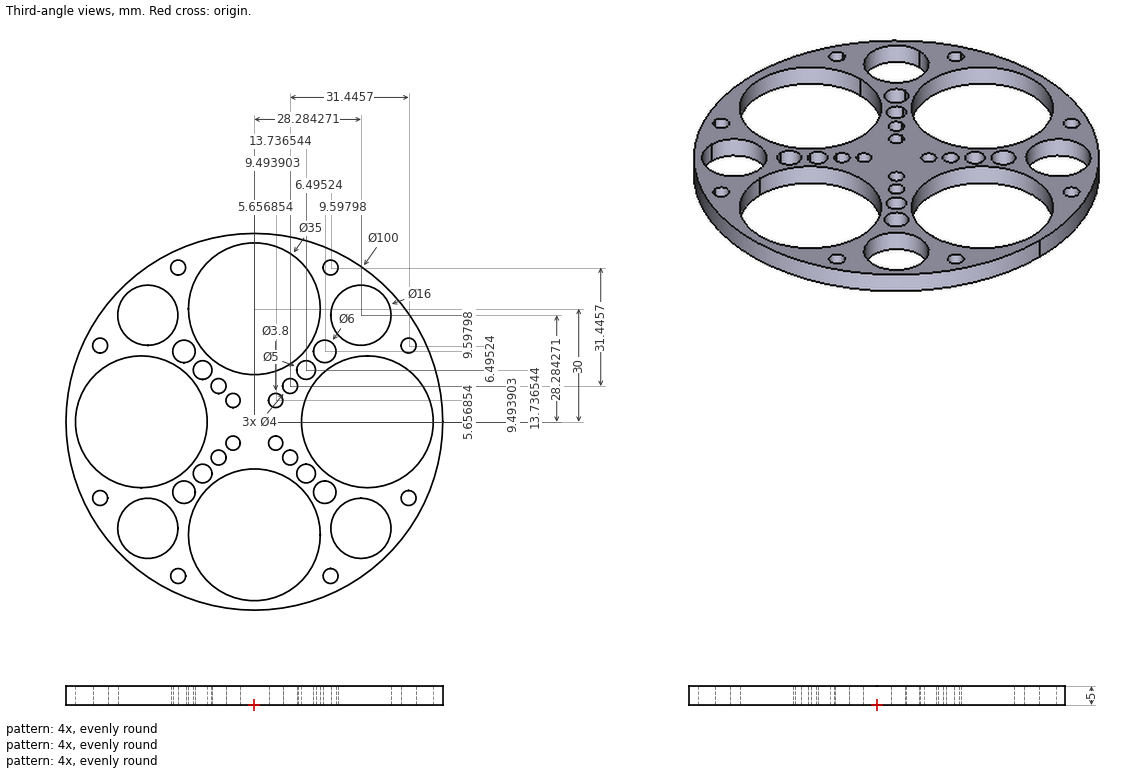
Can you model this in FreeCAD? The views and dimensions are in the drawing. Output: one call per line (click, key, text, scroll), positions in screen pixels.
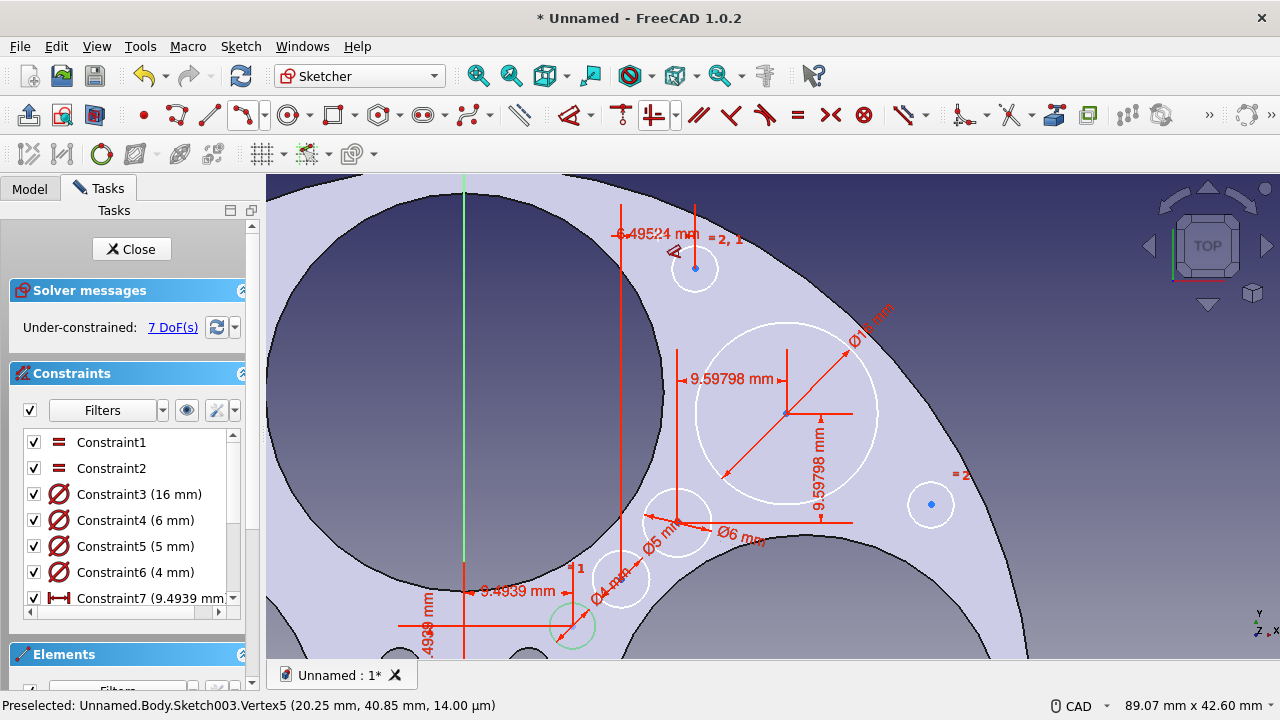
click(573, 626)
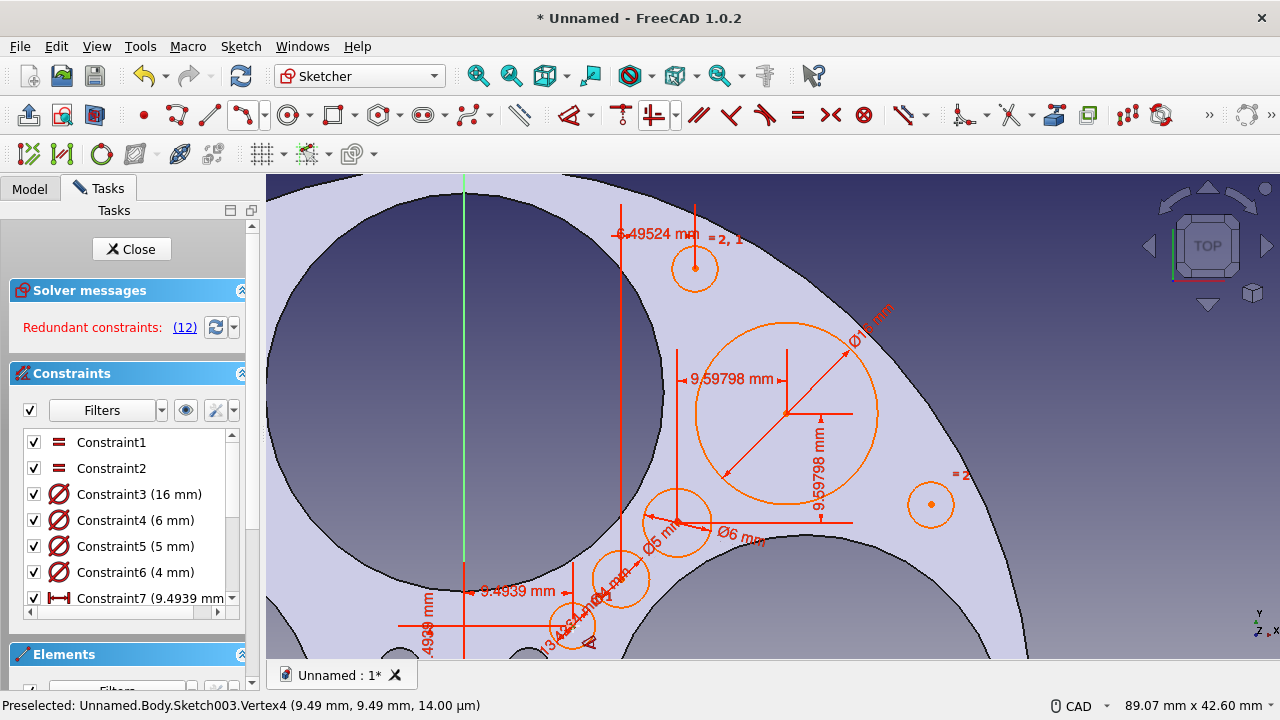
click(695, 269)
click(539, 448)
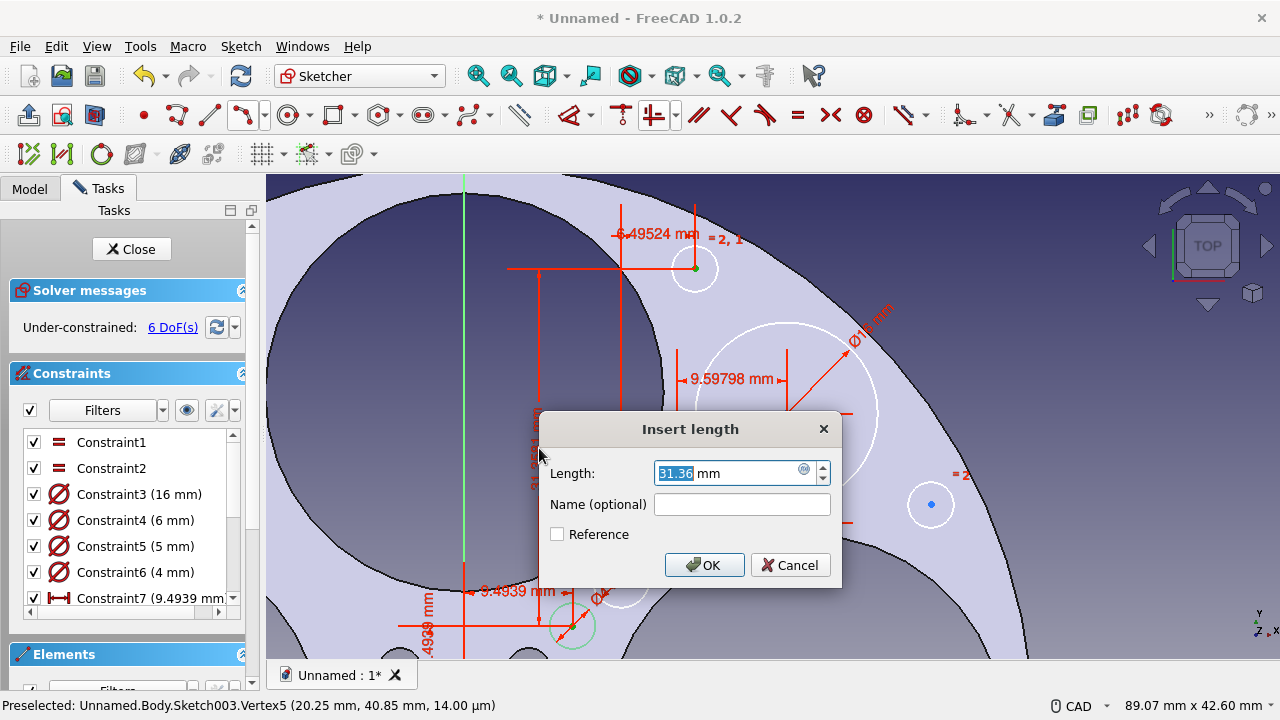
text(31.4457)
key(Return)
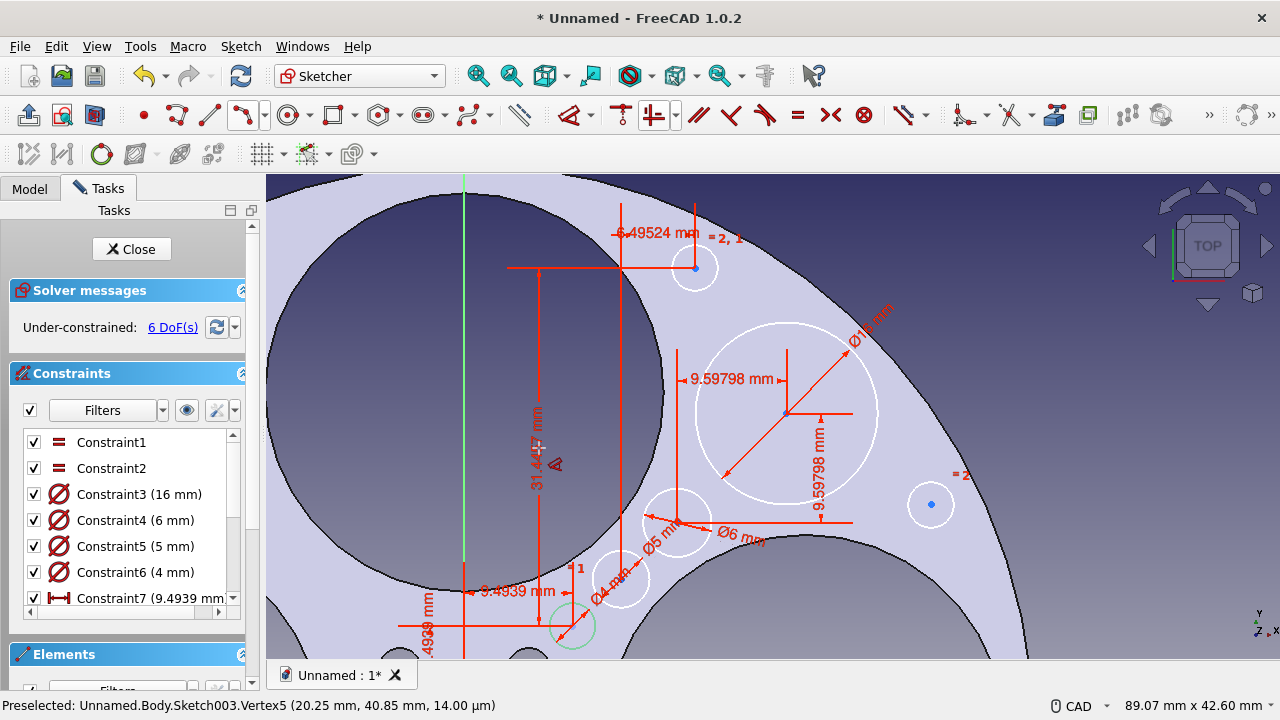
click(573, 626)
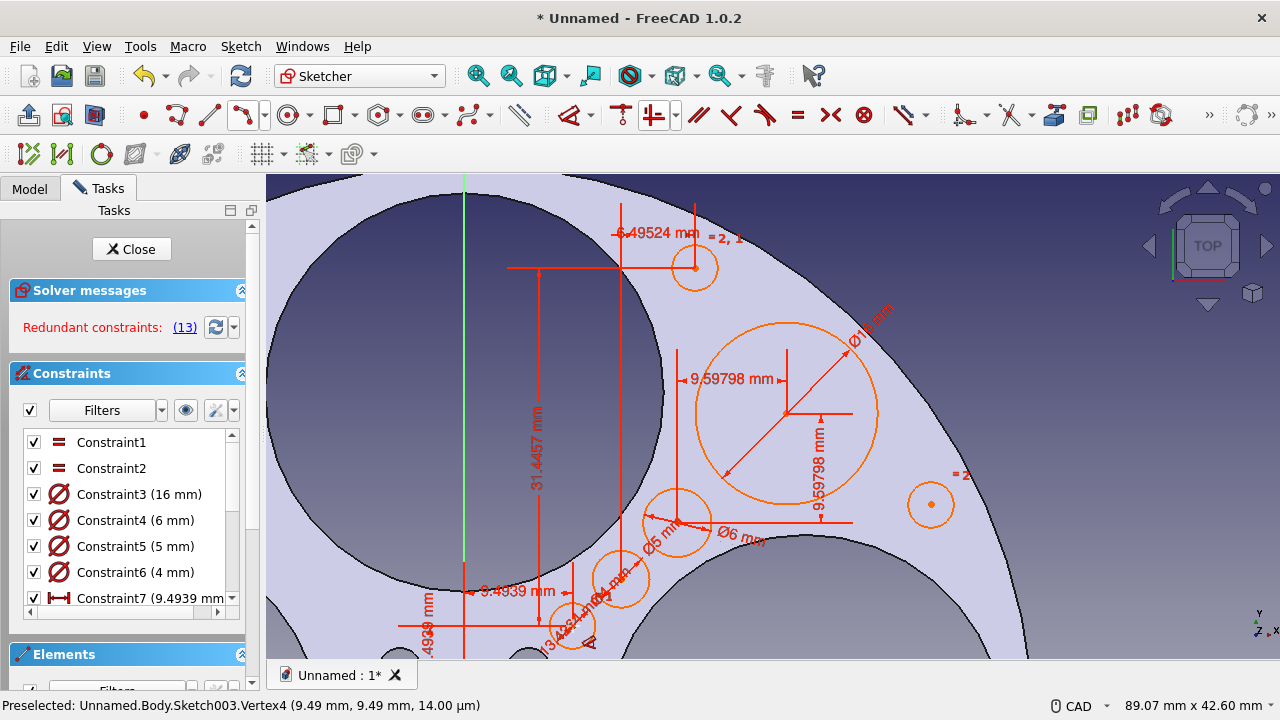
click(931, 505)
click(669, 471)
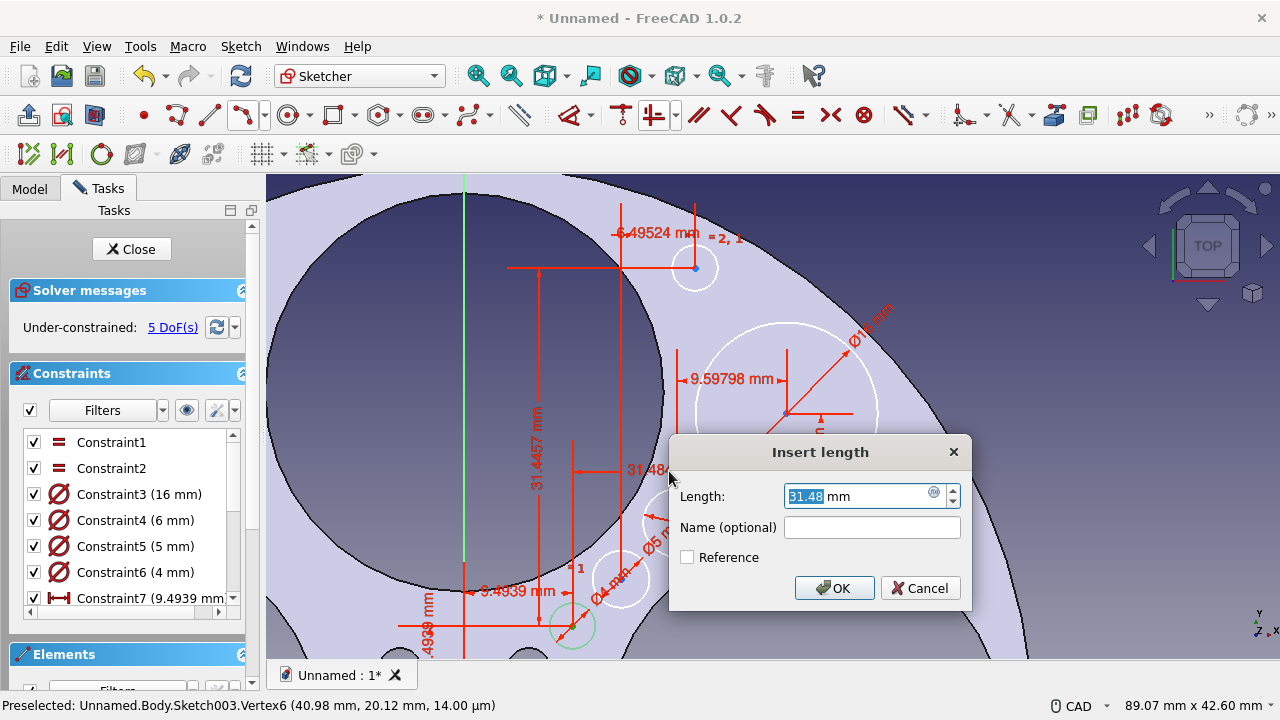
text(31.4457)
key(Return)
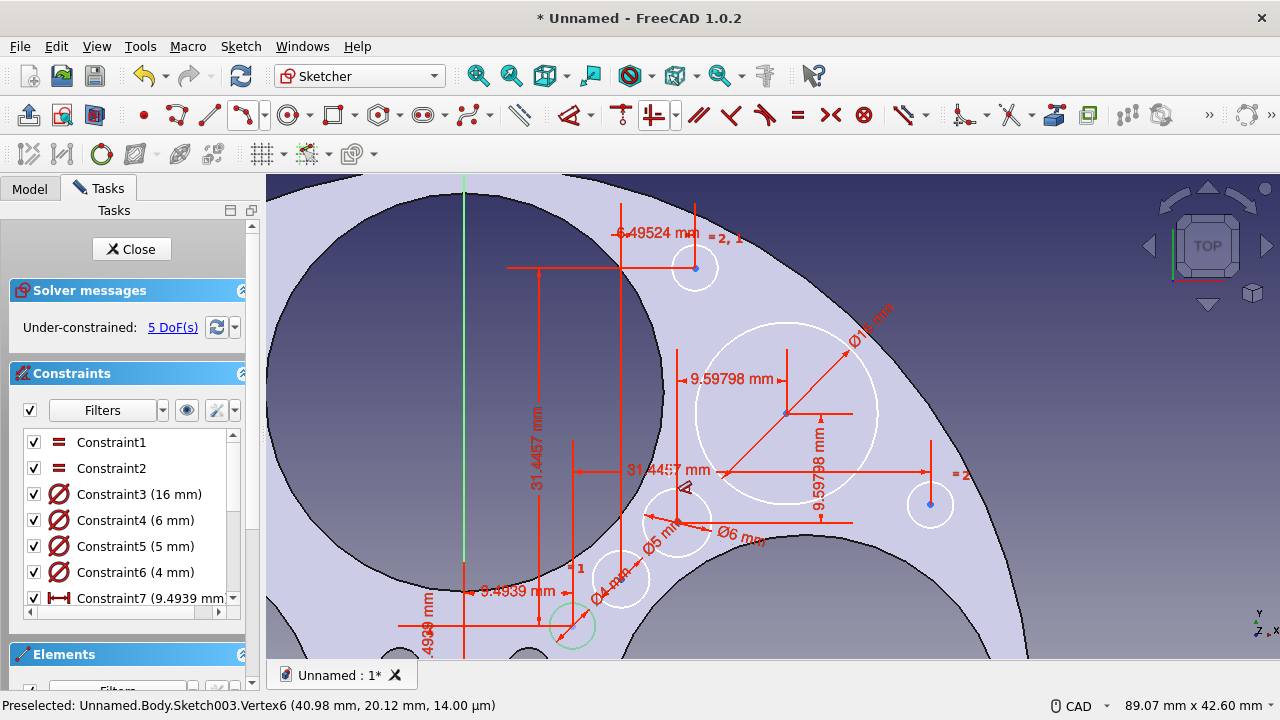
click(621, 579)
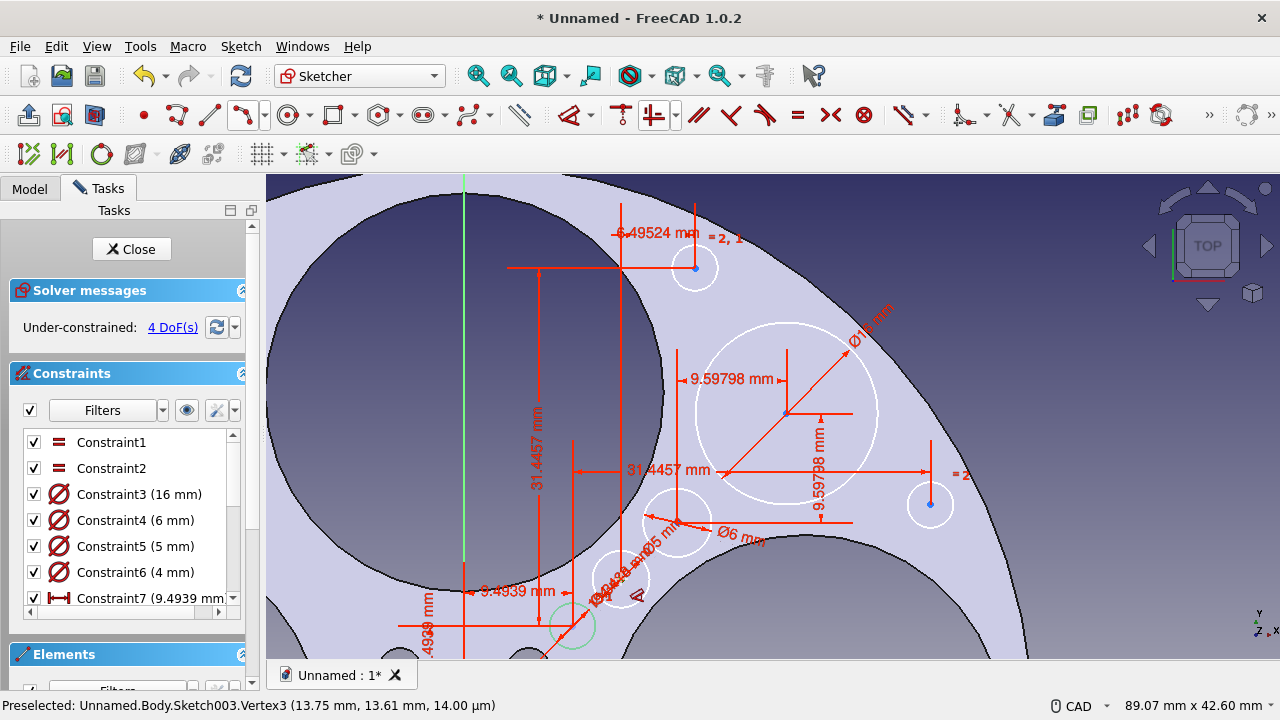
click(931, 505)
click(965, 542)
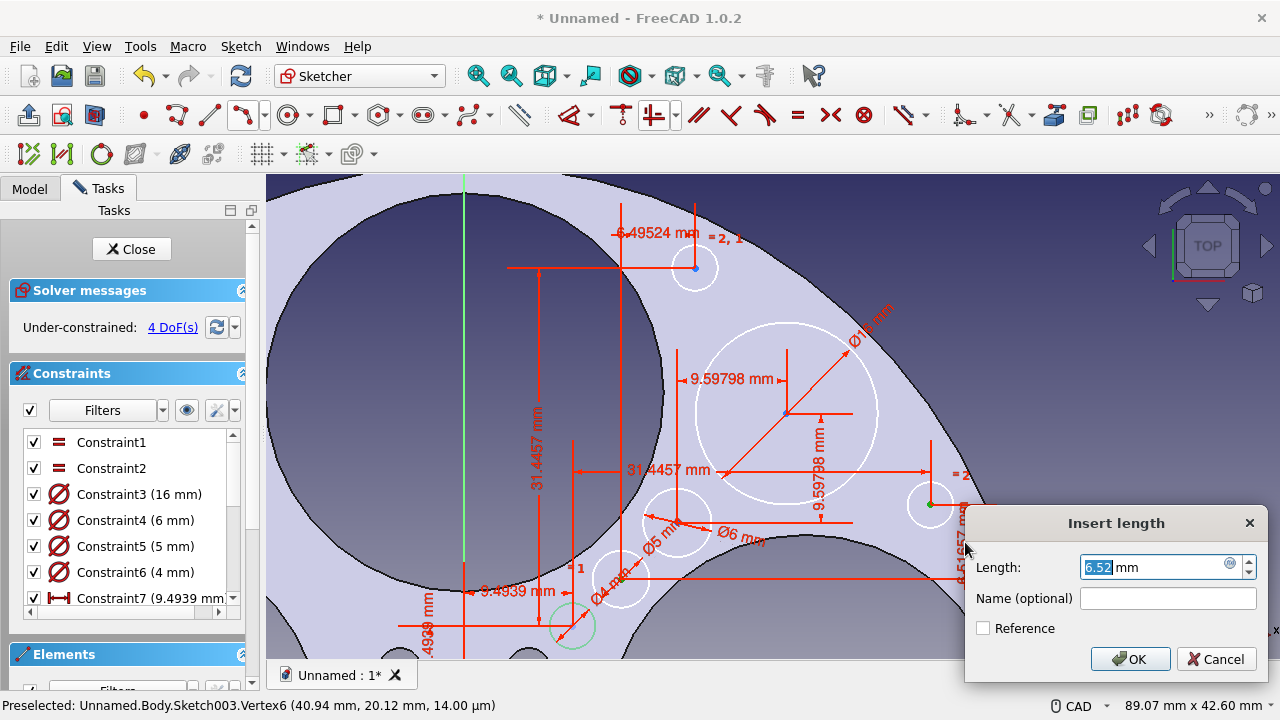
text(6.49524)
key(Return)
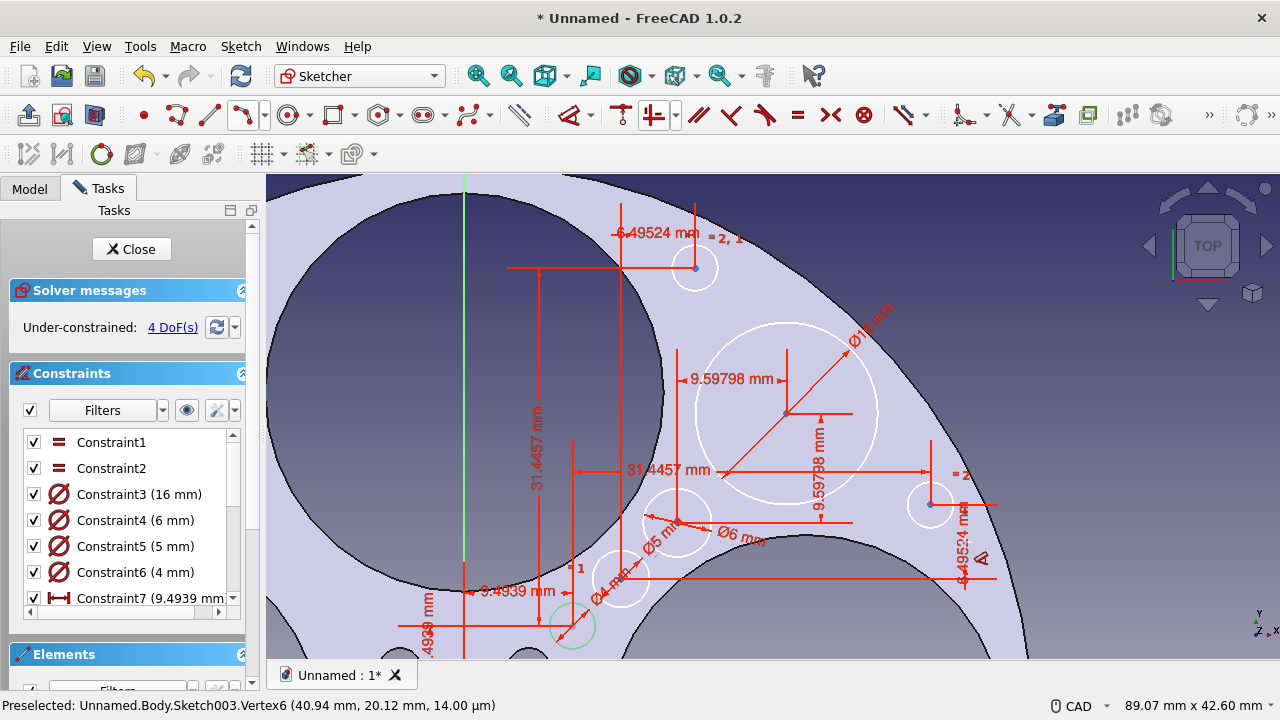
click(787, 414)
click(626, 380)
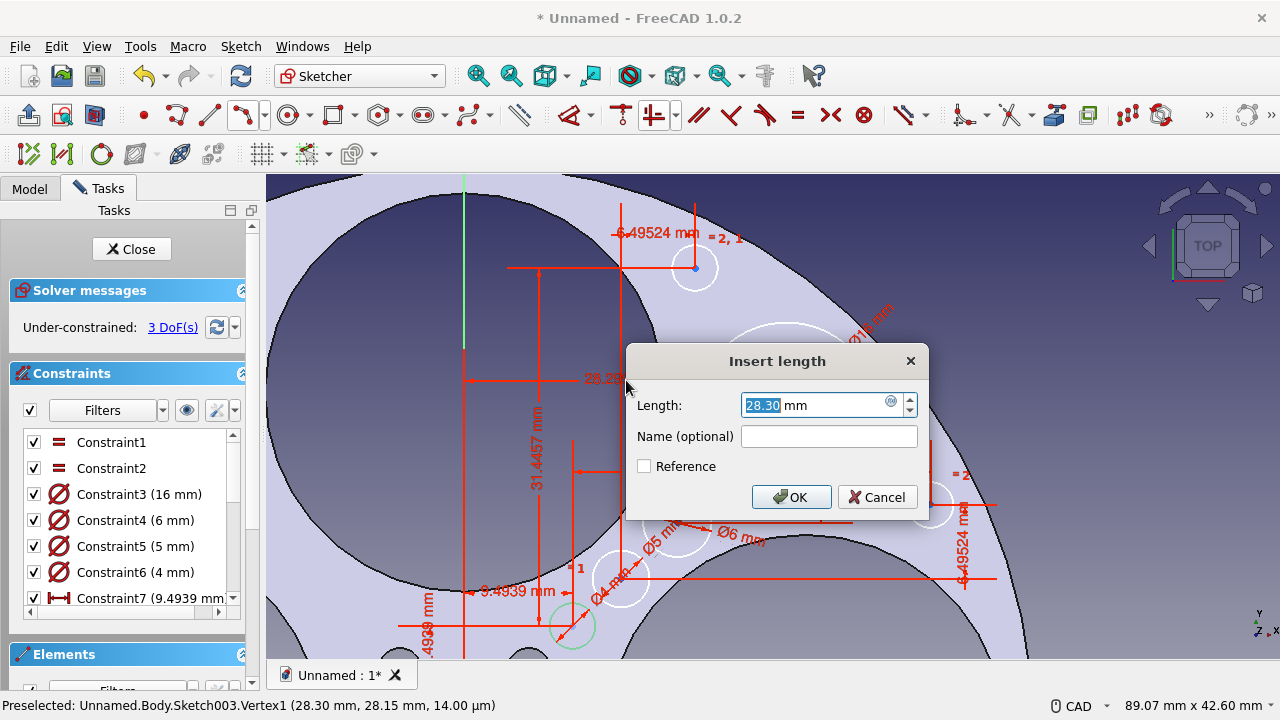
text(28.284271)
key(Return)